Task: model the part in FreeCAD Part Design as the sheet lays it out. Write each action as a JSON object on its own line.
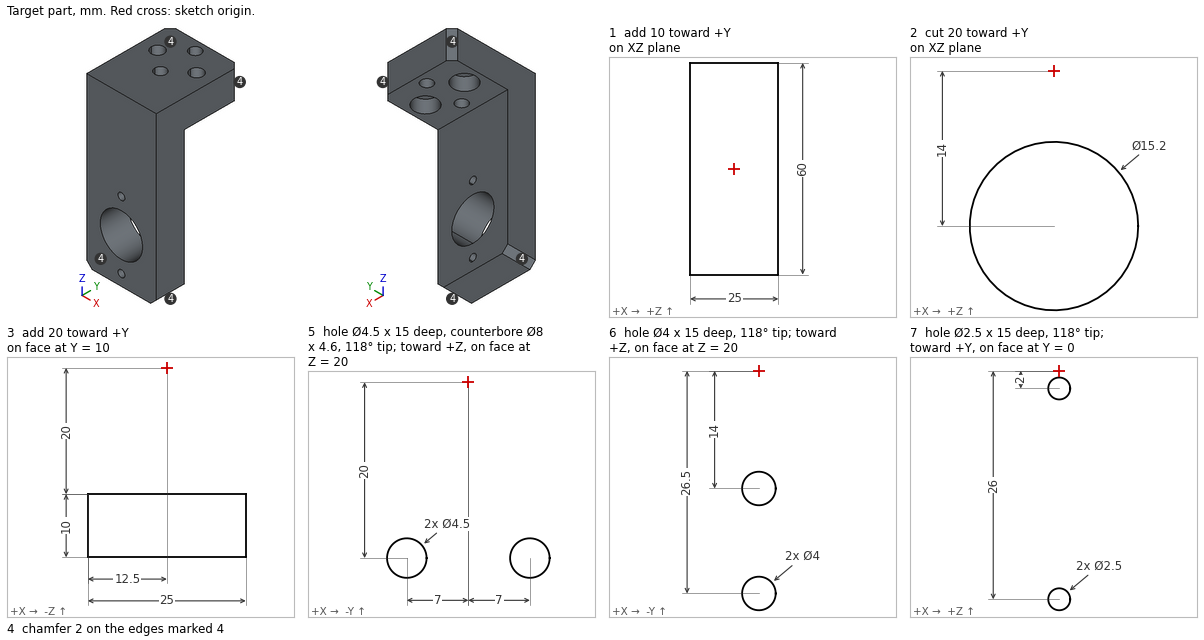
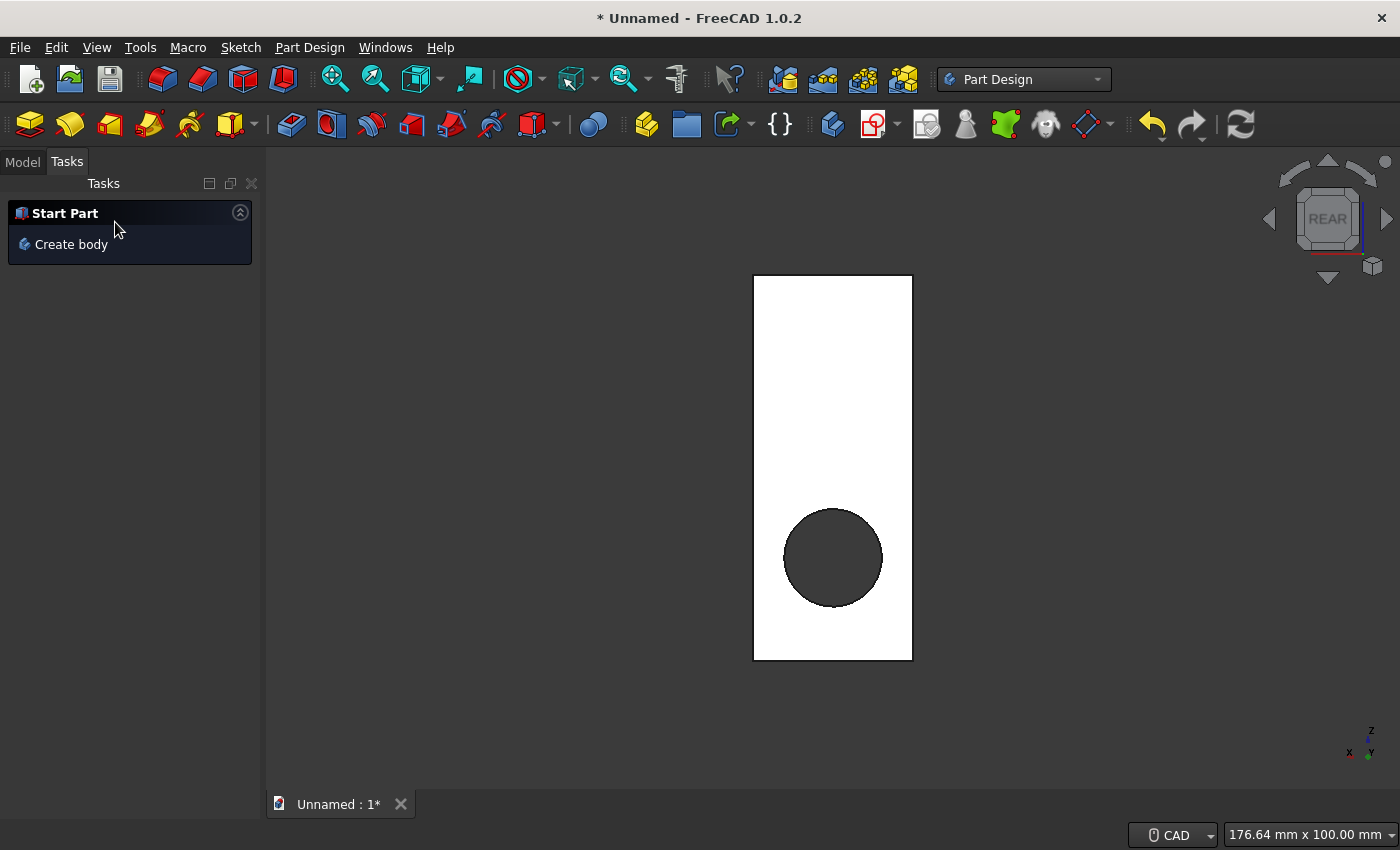
{"action": "left_click", "coordinate": [833, 357]}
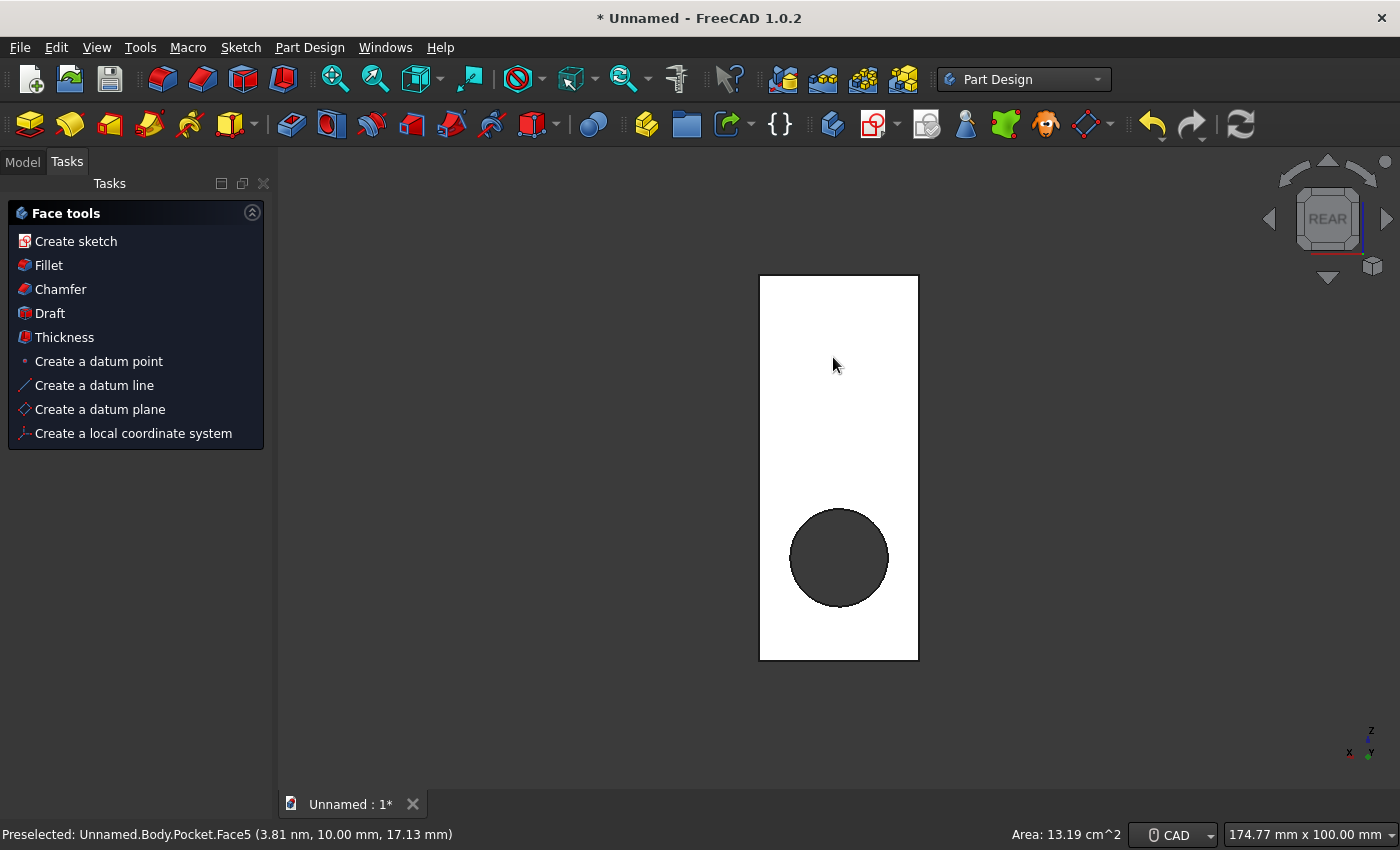
{"action": "left_click", "coordinate": [874, 124]}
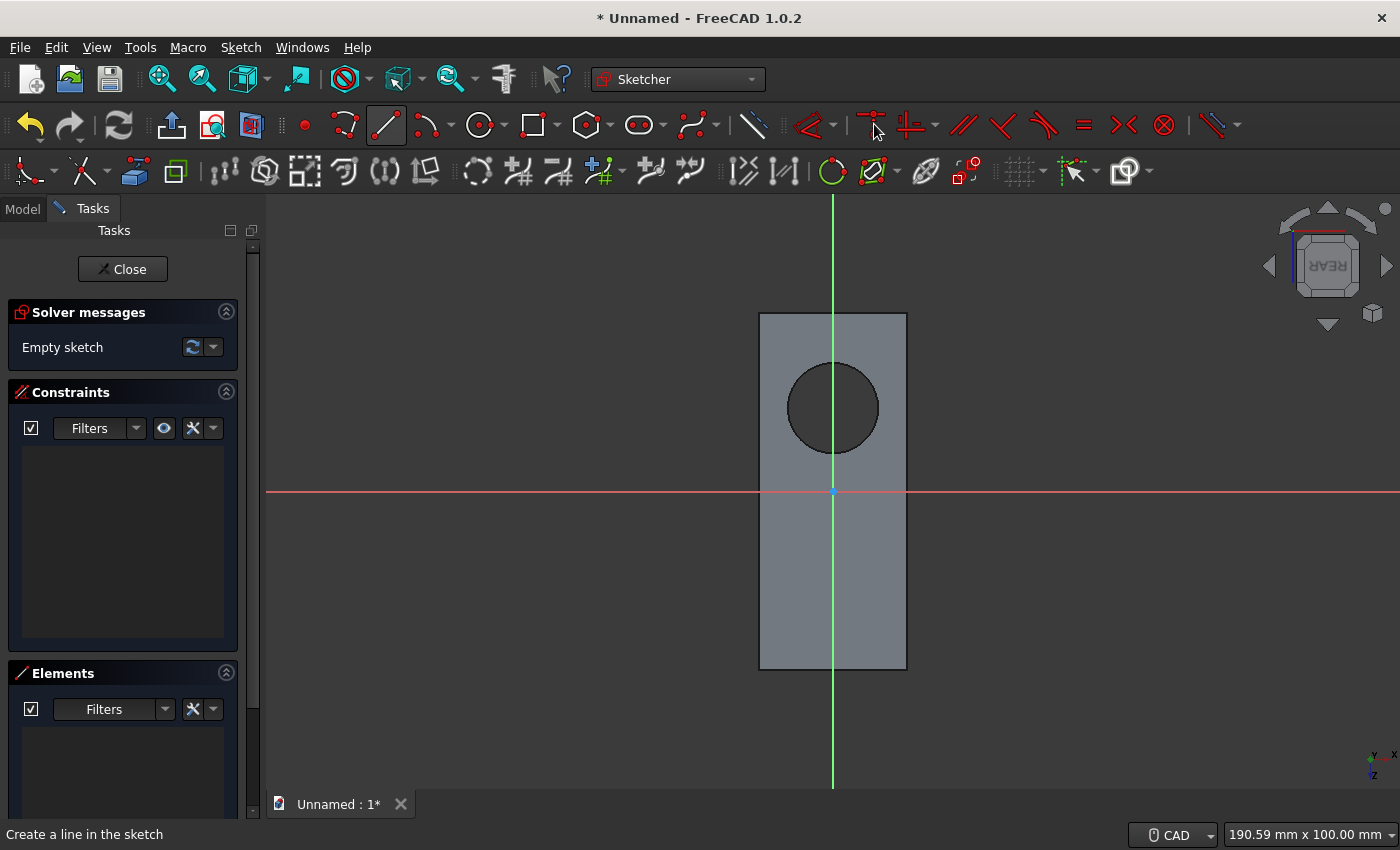
{"action": "scroll", "coordinate": [889, 654], "scroll_direction": "up", "scroll_amount": 4}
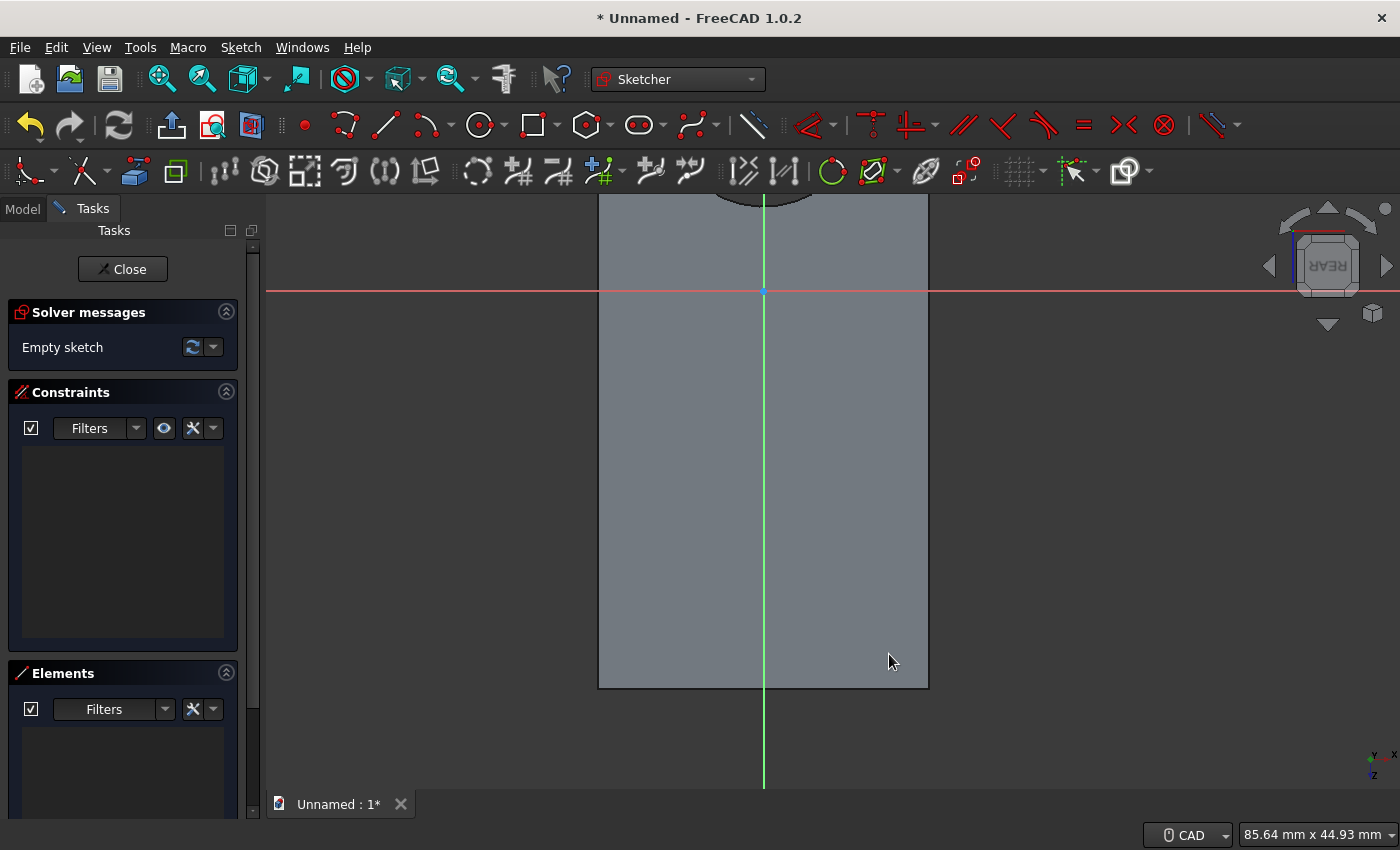
{"action": "key", "text": "g r"}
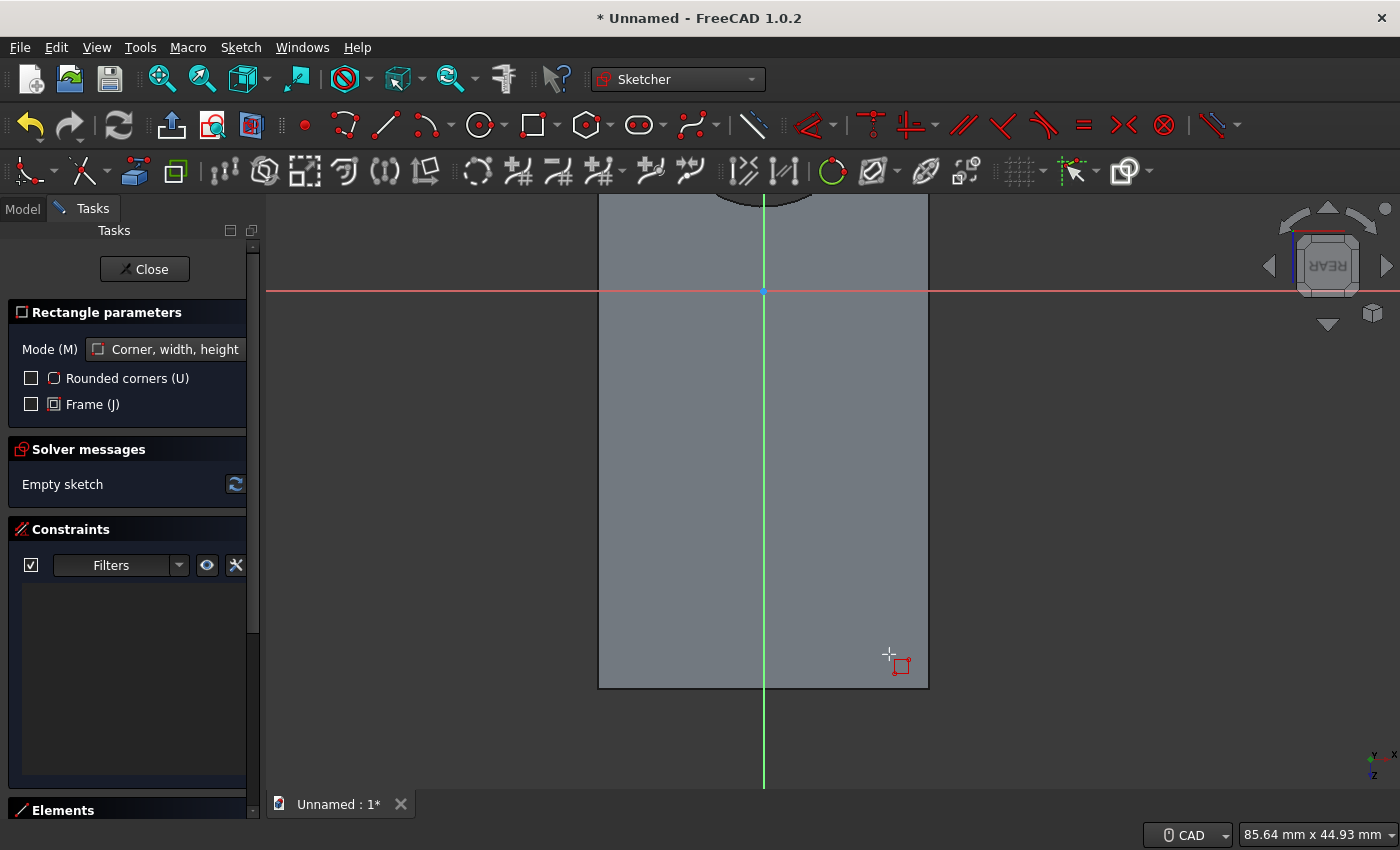
{"action": "left_click", "coordinate": [598, 556]}
{"action": "left_click", "coordinate": [929, 689]}
{"action": "key", "text": "Escape"}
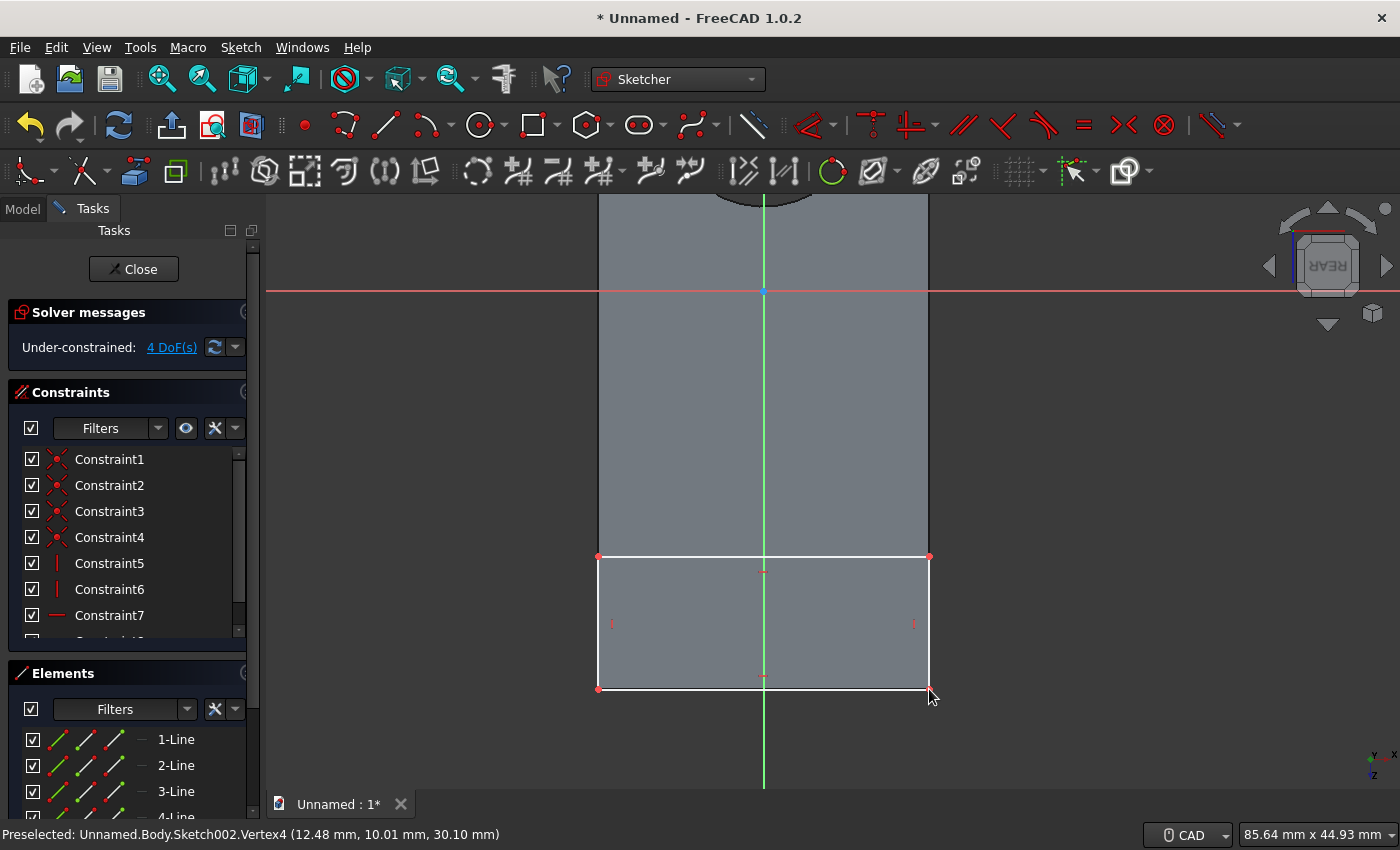
{"action": "key", "text": "d"}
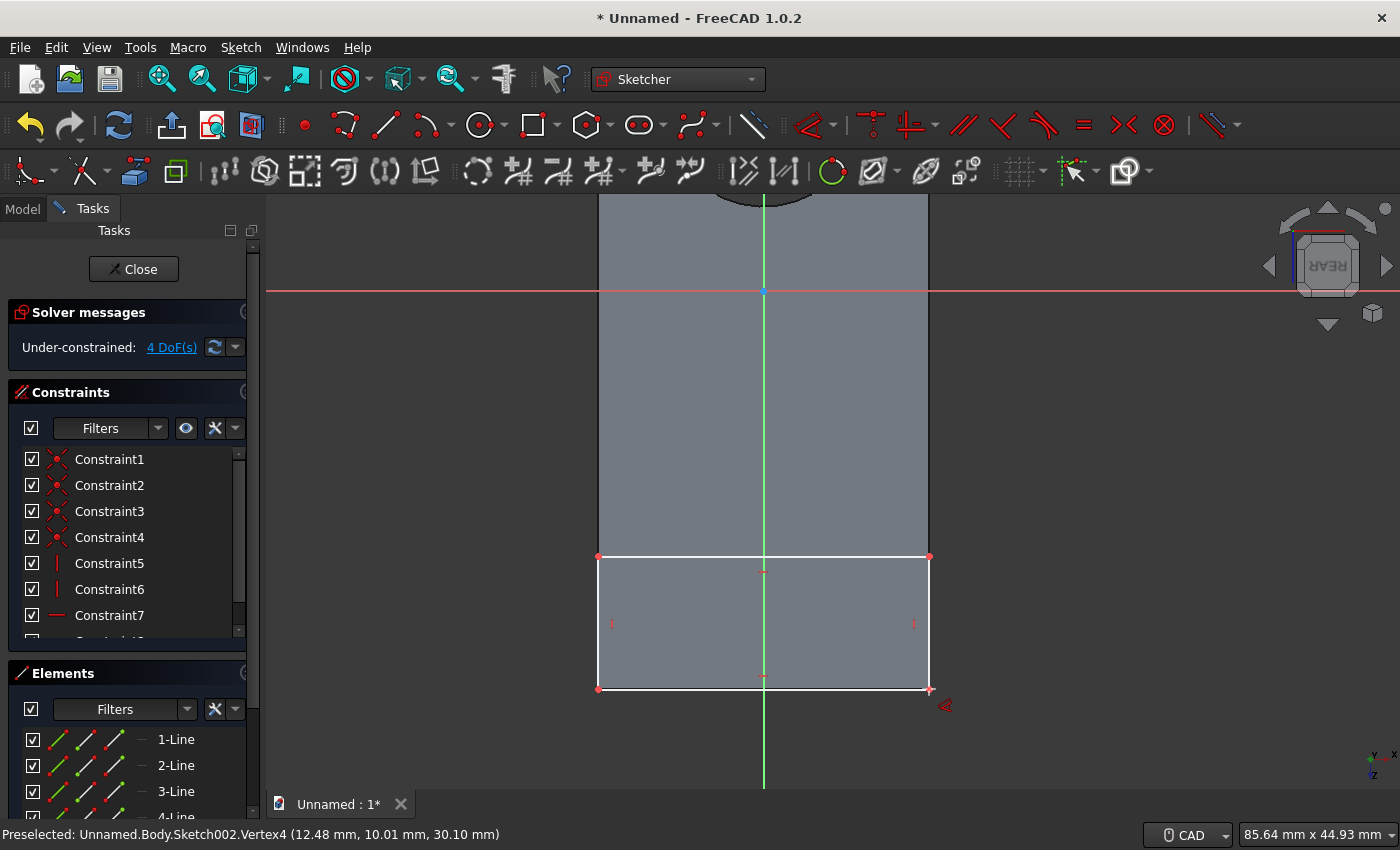
{"action": "left_click", "coordinate": [598, 597]}
{"action": "left_click", "coordinate": [564, 623]}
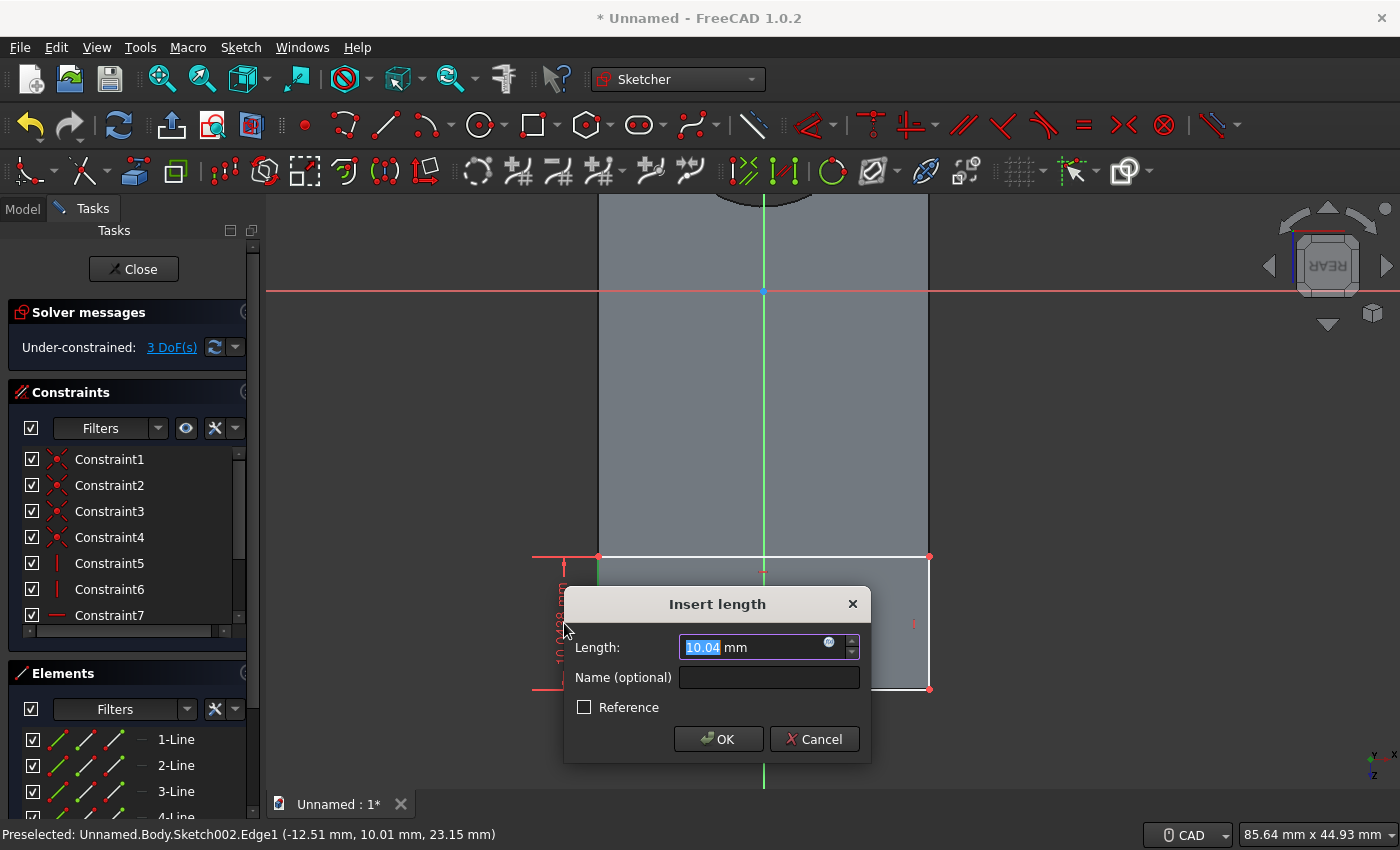
{"action": "type", "text": "10"}
{"action": "key", "text": "Return"}